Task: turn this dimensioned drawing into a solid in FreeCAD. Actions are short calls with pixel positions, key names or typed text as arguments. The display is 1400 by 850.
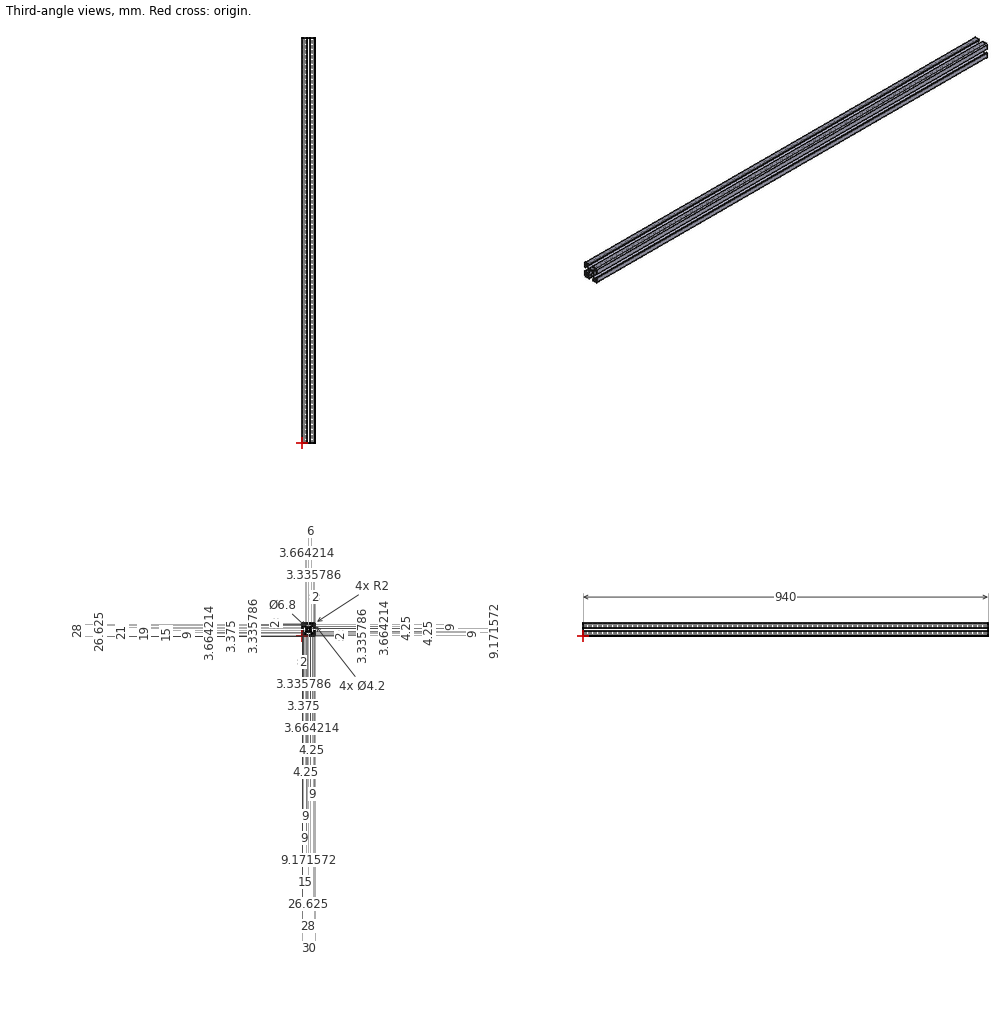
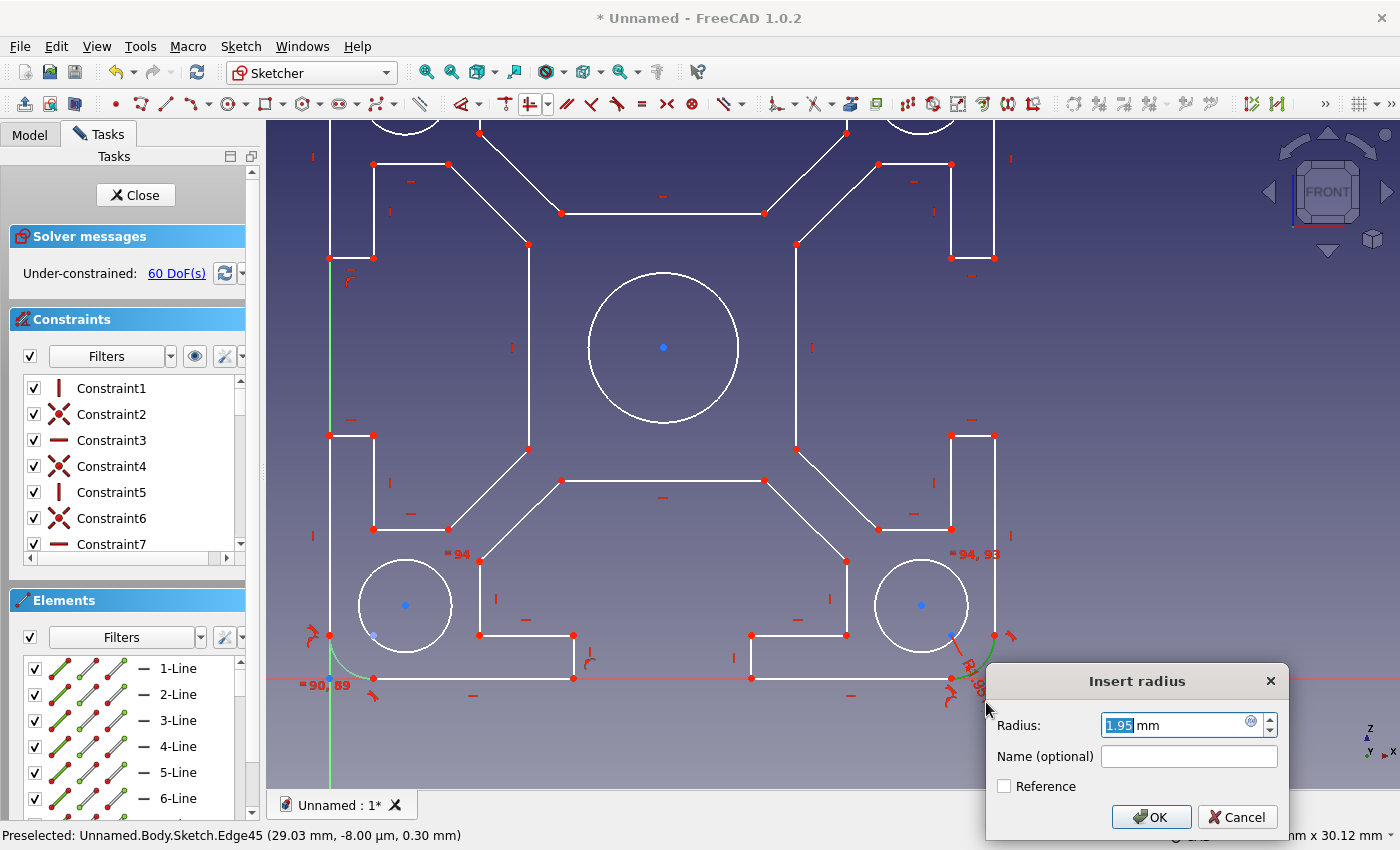
text(2)
key(Return)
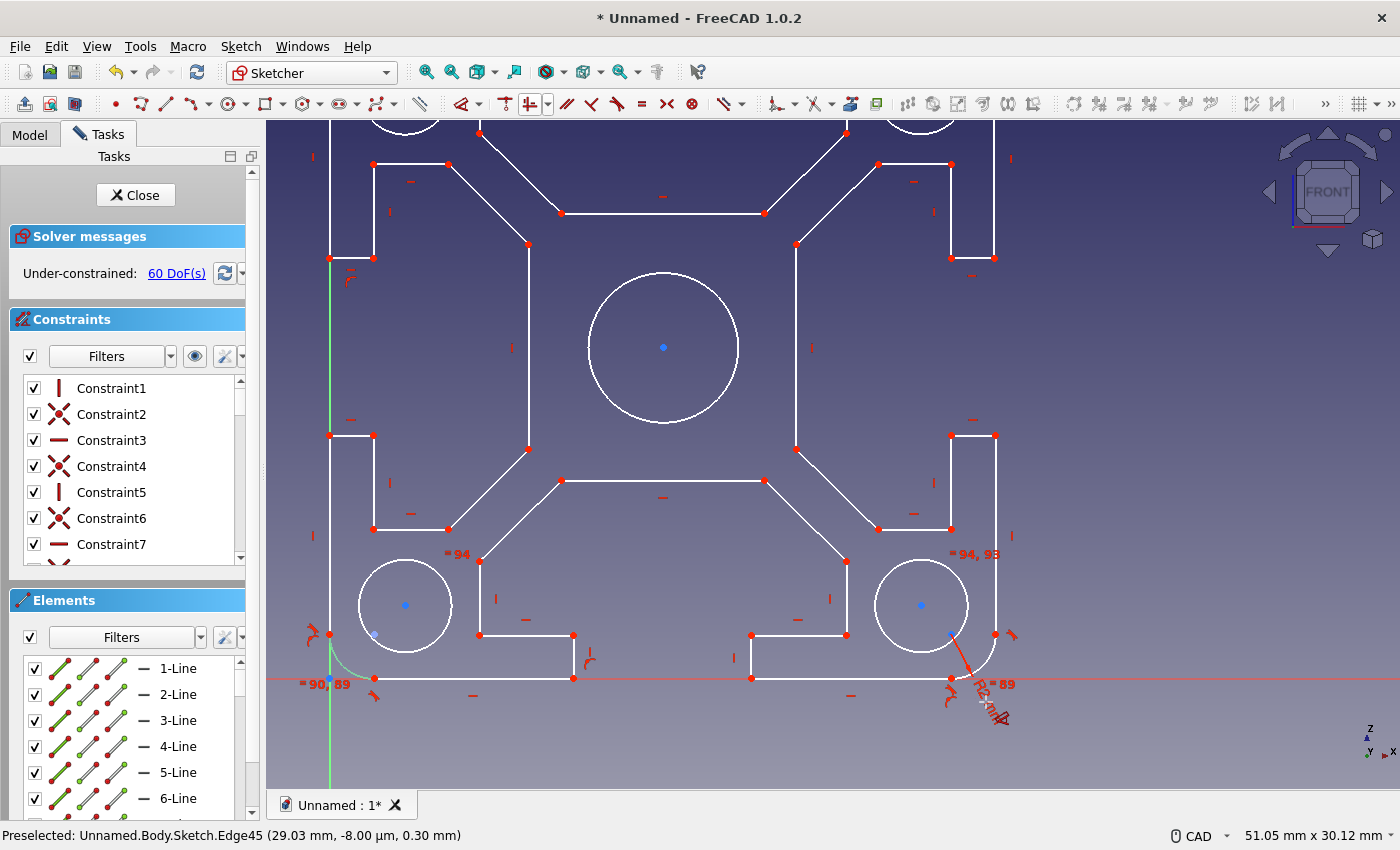
scroll(971, 676, down, 2)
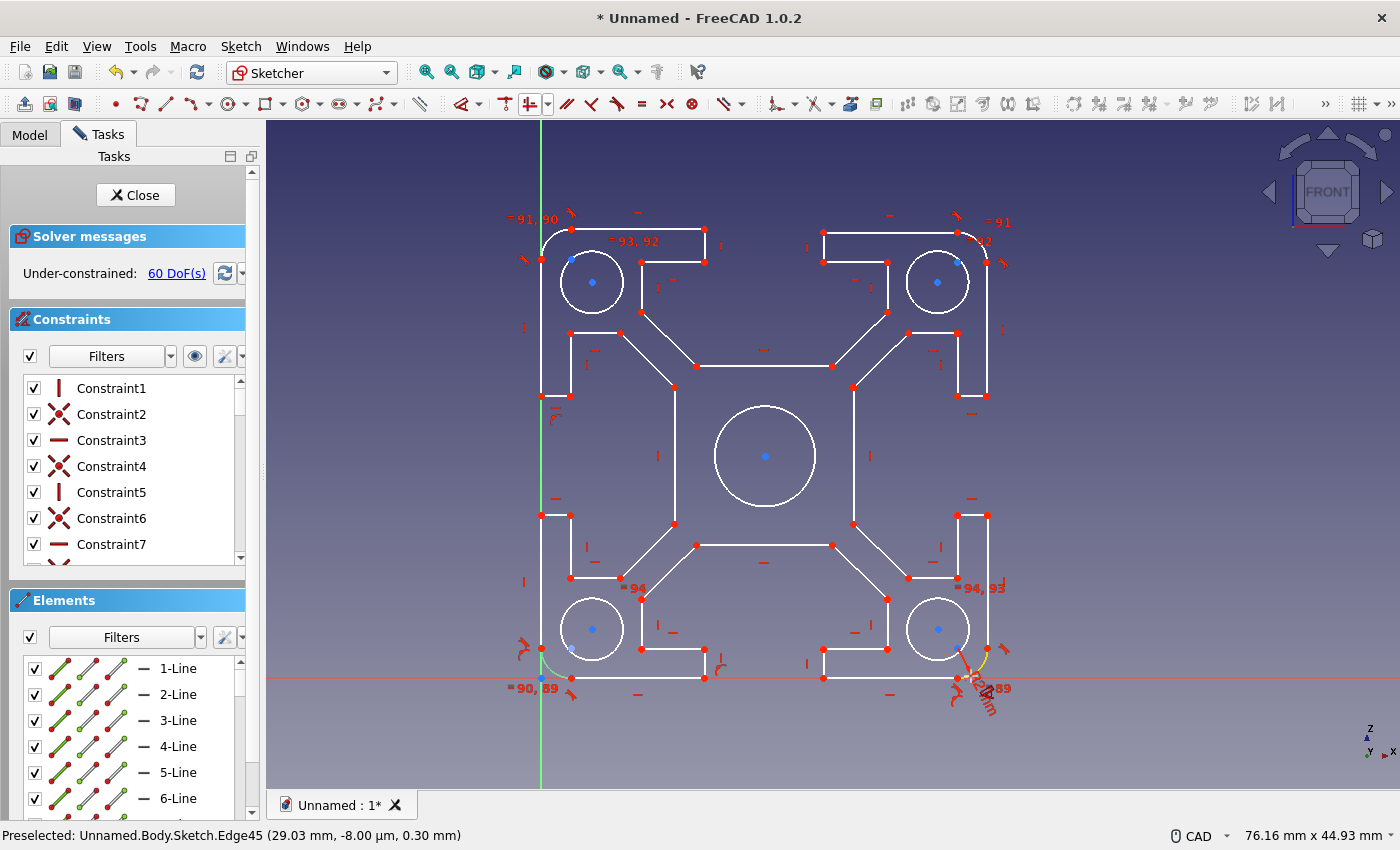
click(916, 260)
click(914, 199)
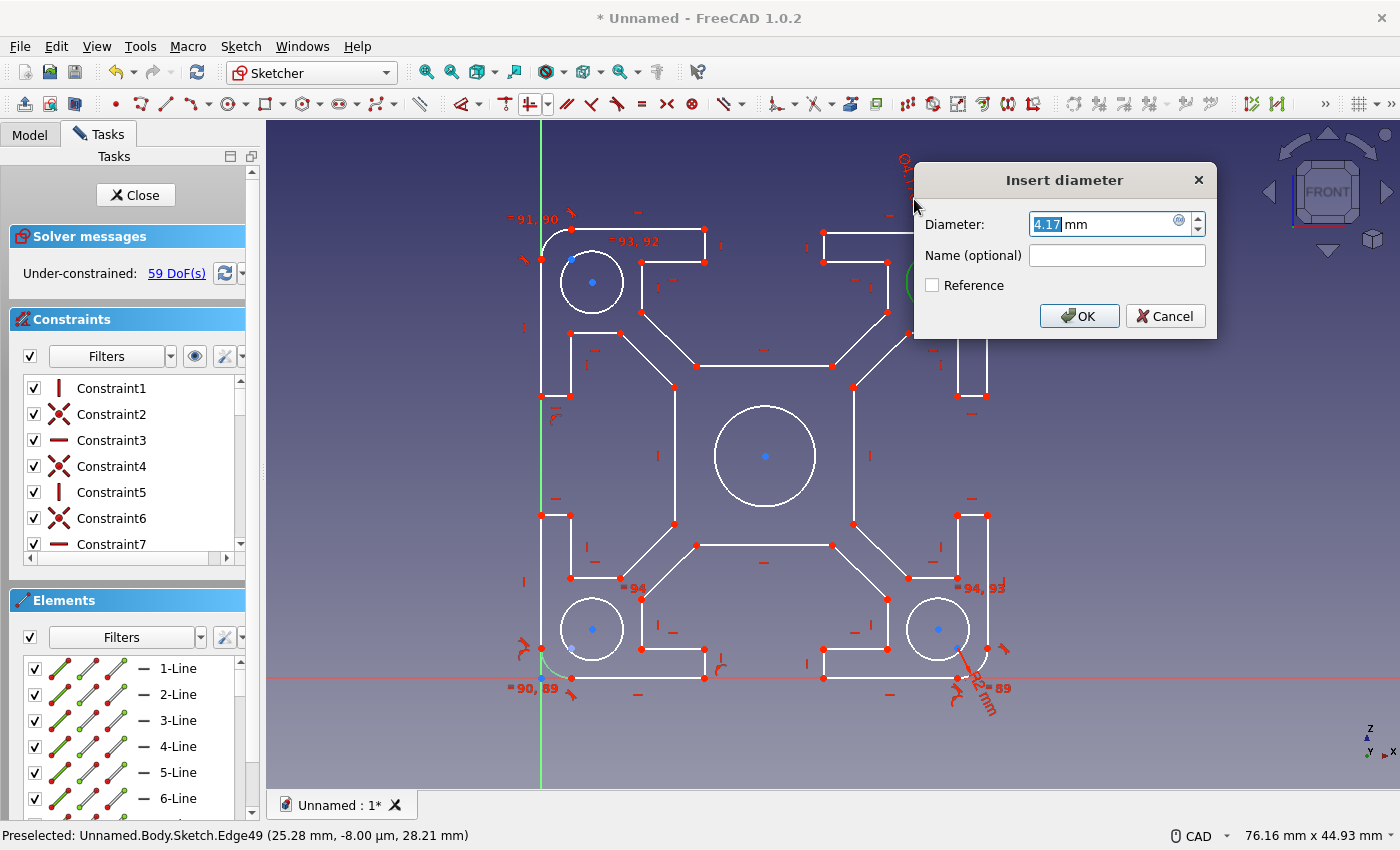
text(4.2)
key(Return)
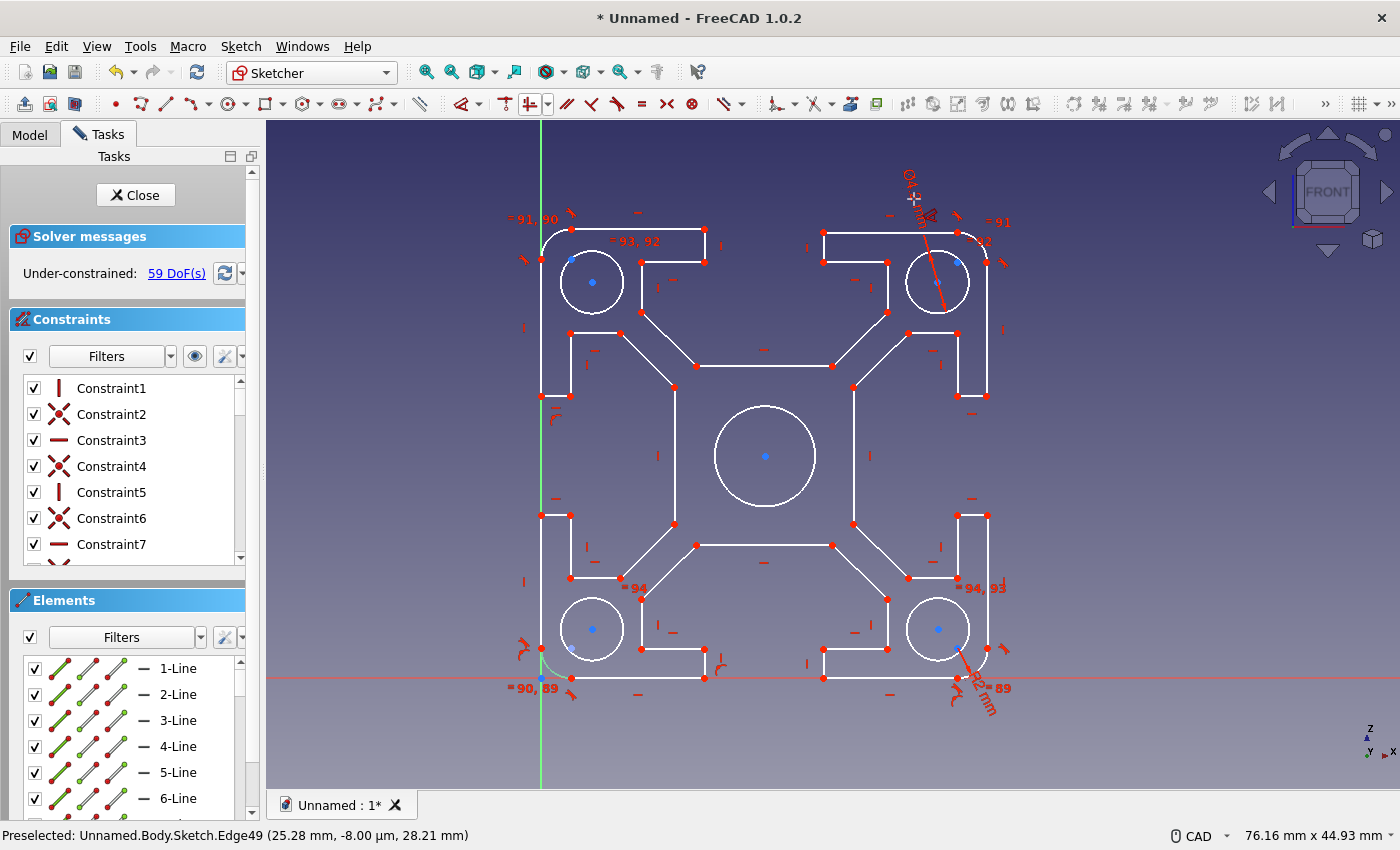
click(800, 421)
click(823, 398)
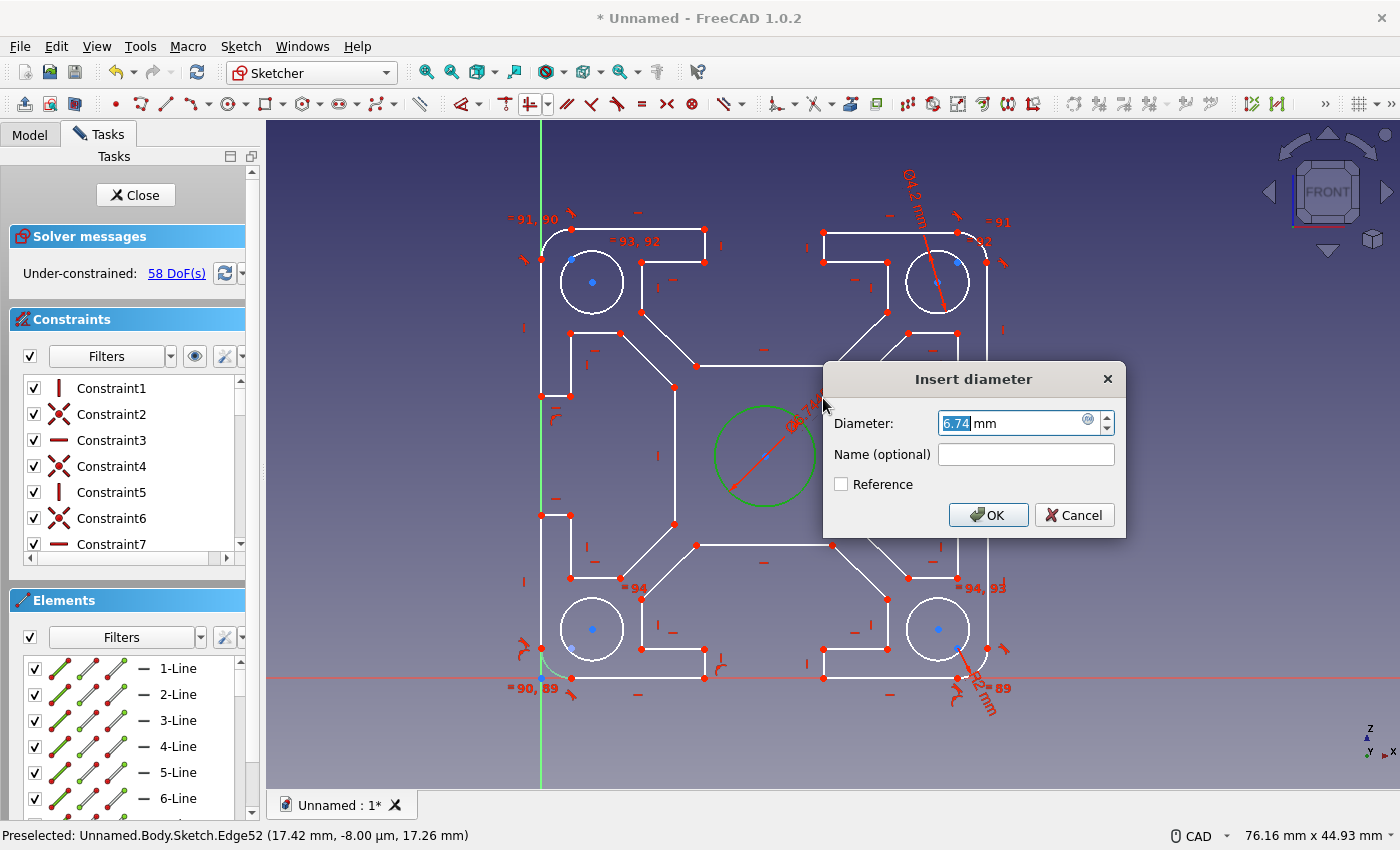
text(6.8)
key(Return)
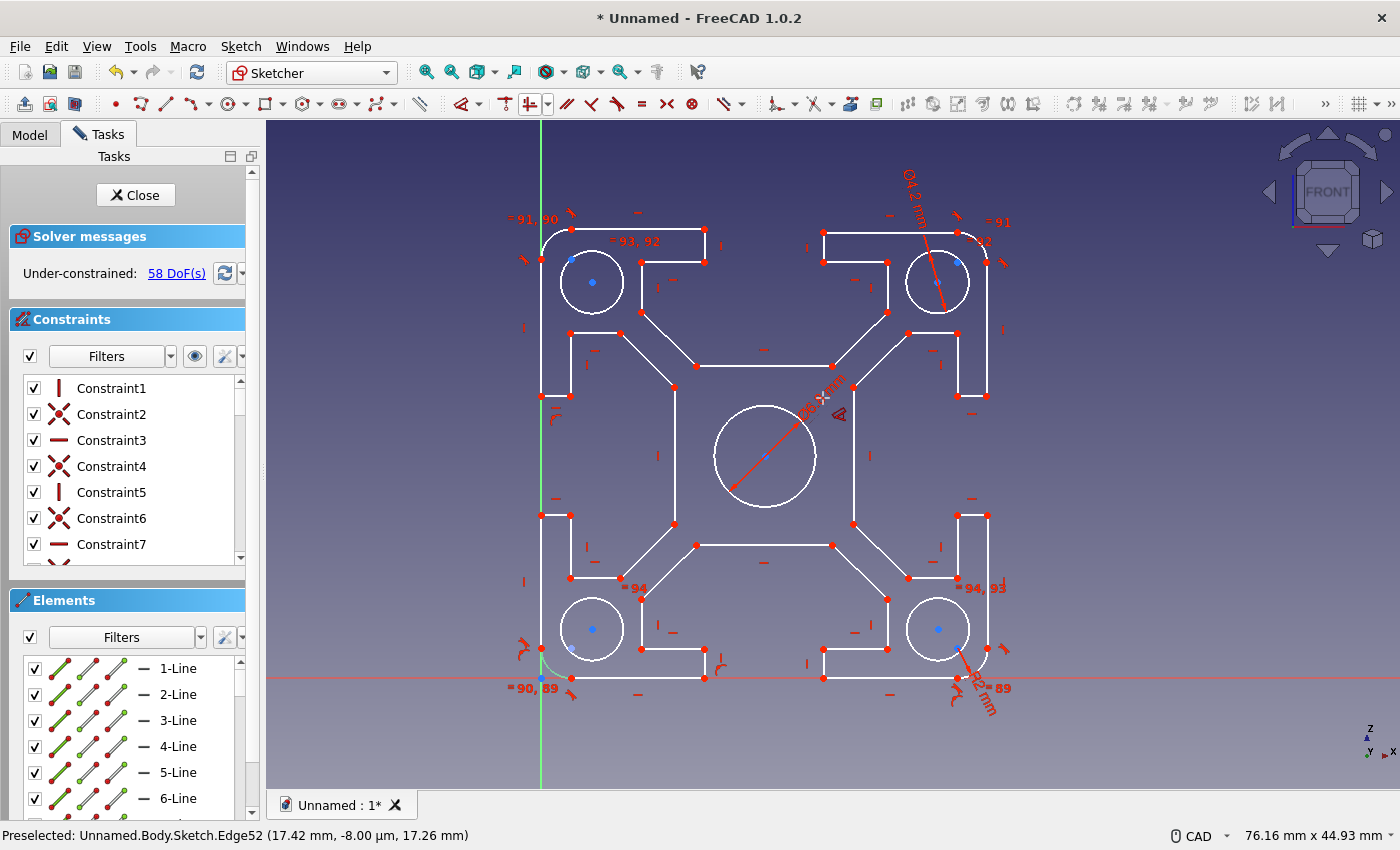
click(987, 303)
click(1021, 329)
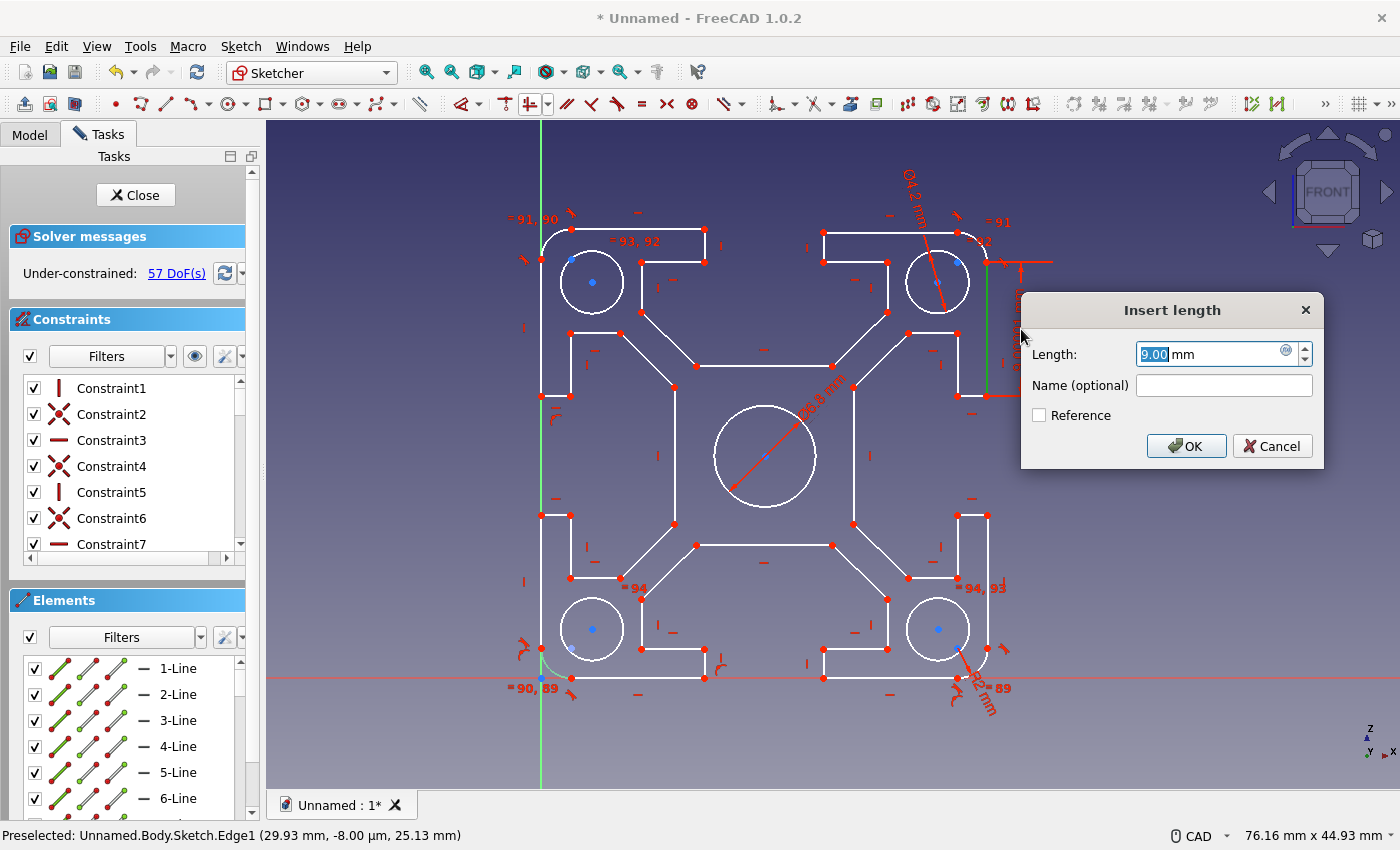
text(9)
key(Return)